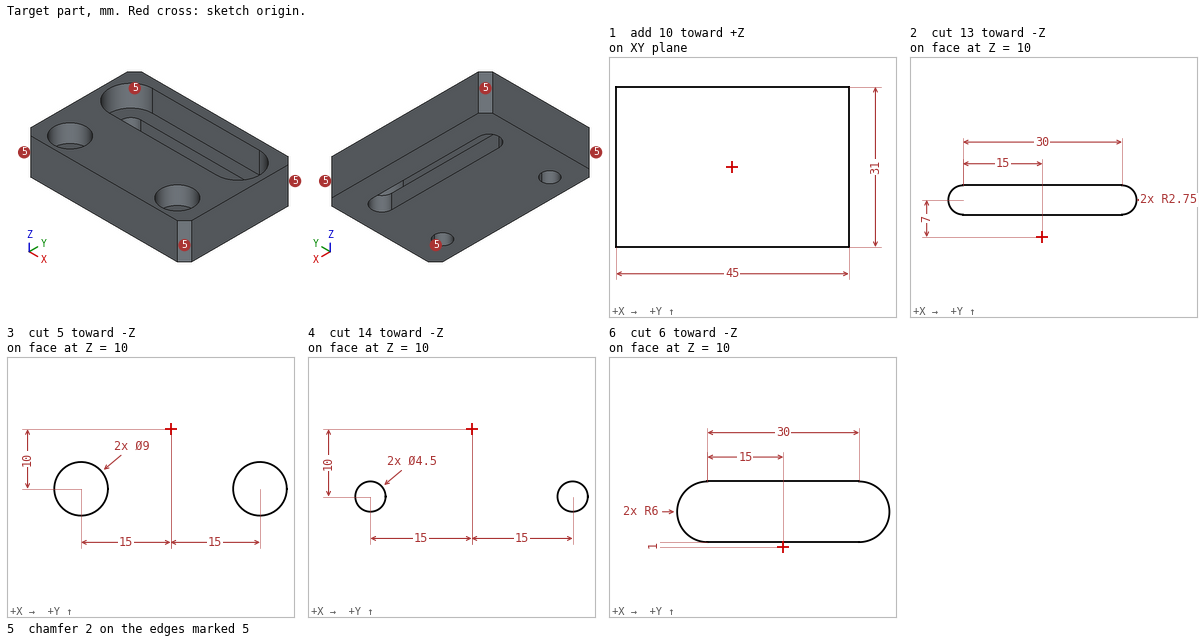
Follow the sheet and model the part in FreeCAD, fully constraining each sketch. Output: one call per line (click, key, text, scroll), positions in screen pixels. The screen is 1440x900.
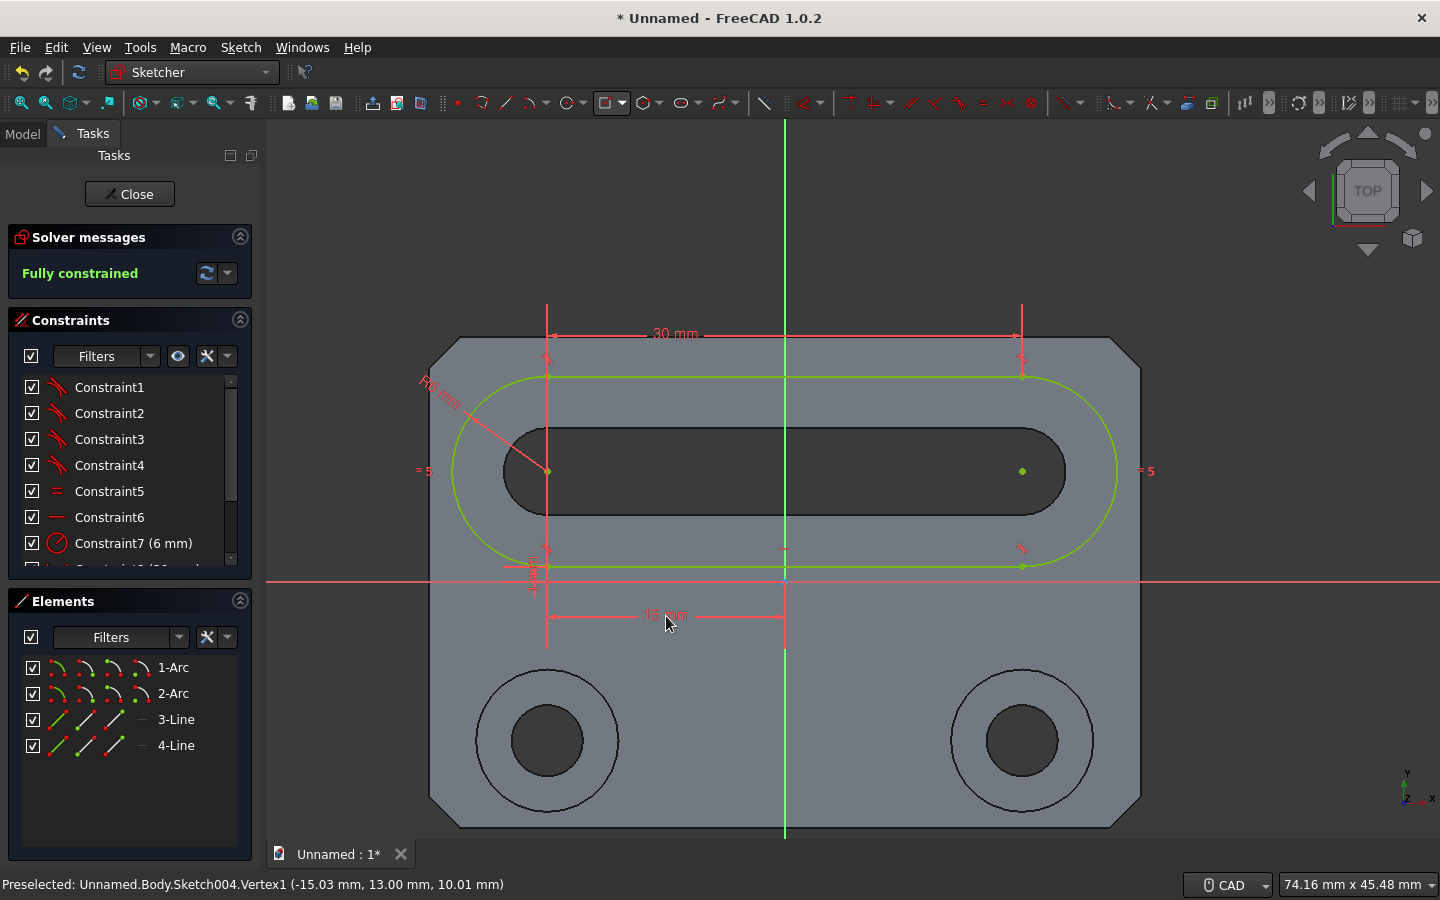
click(130, 194)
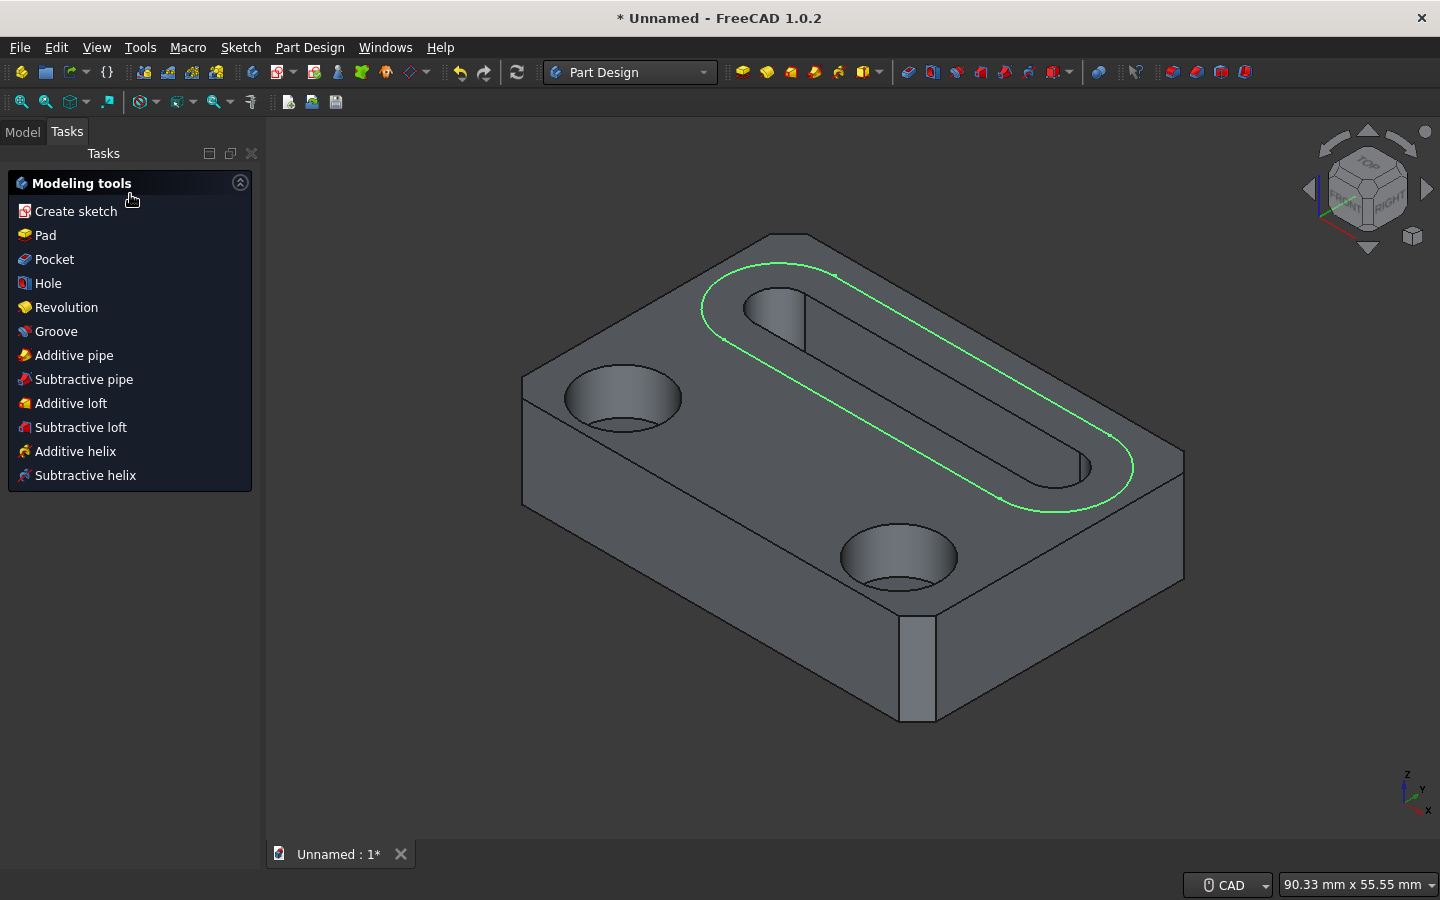
click(910, 72)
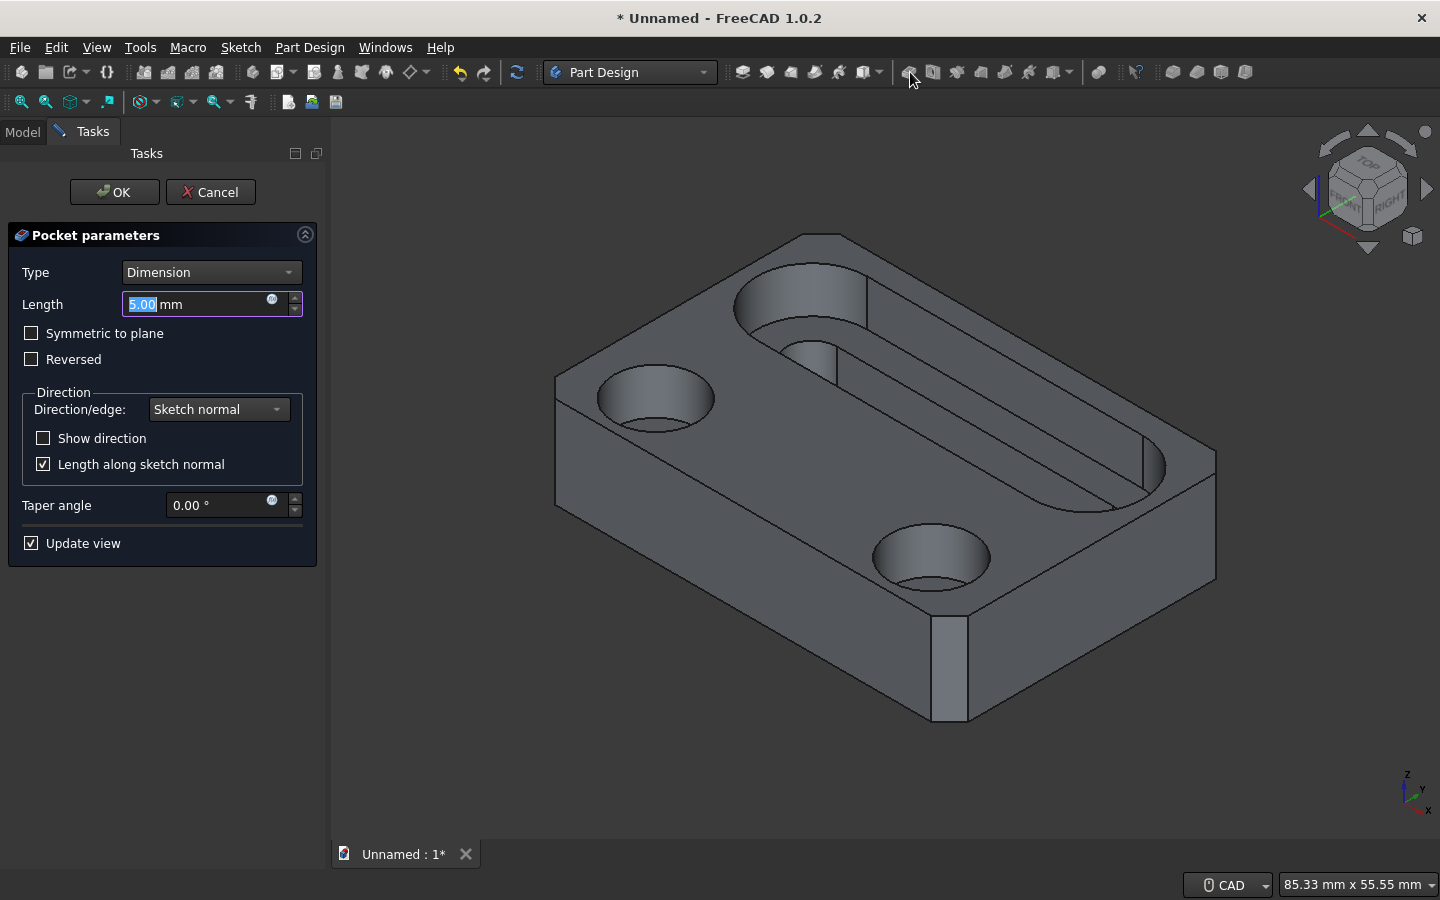
text(6)
key(Tab)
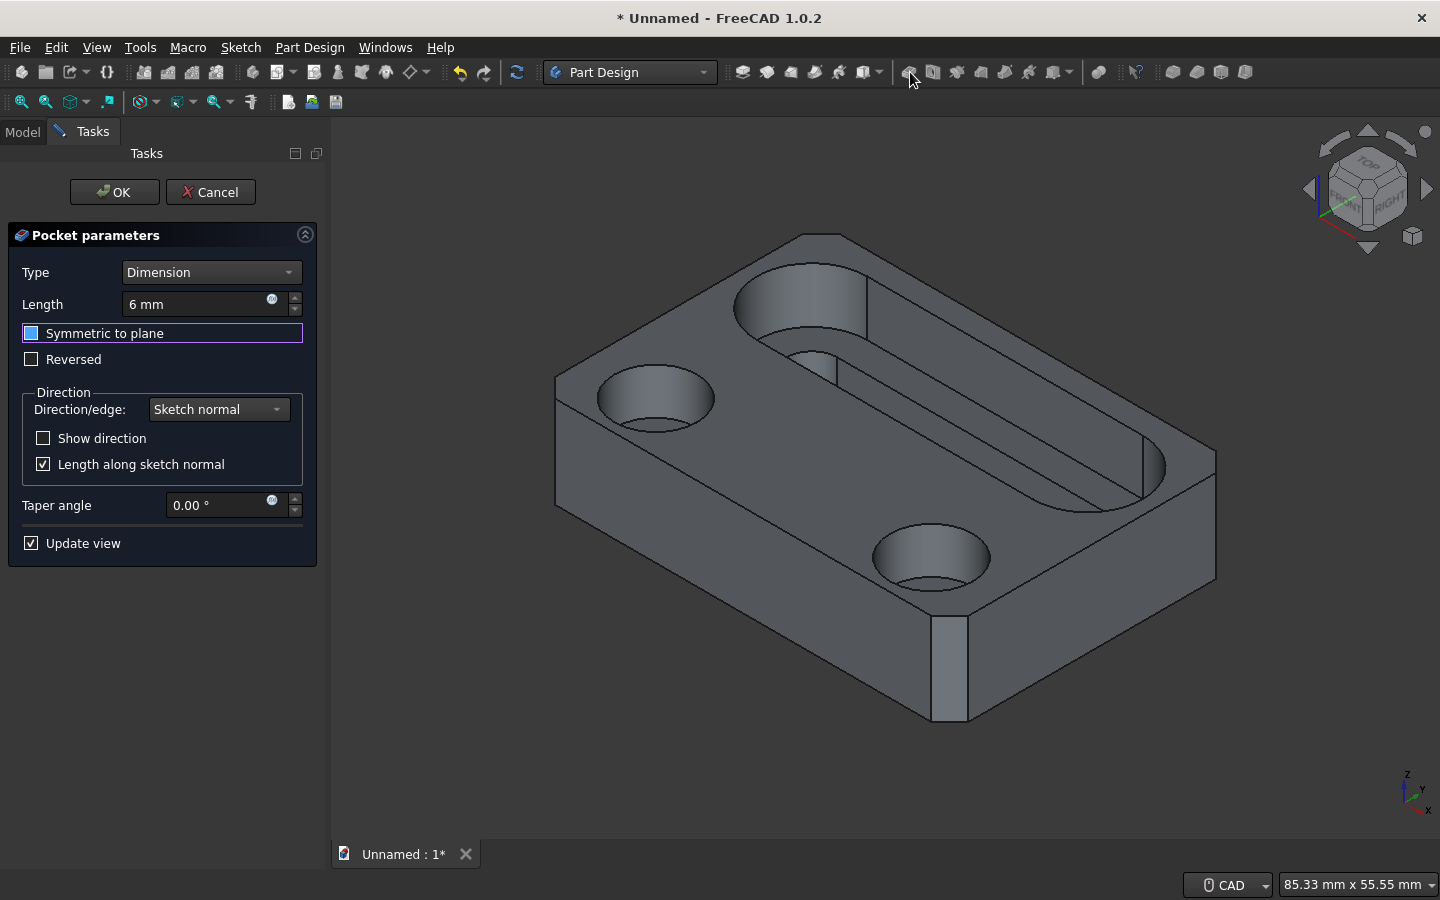
click(115, 192)